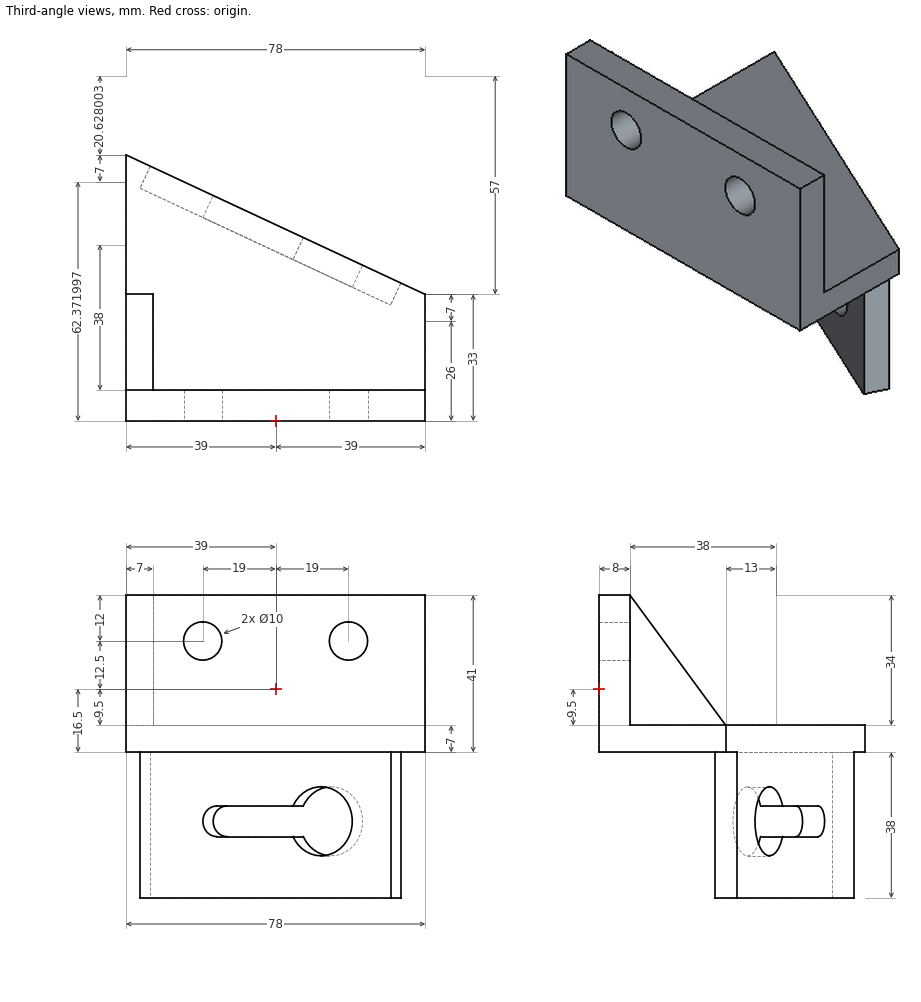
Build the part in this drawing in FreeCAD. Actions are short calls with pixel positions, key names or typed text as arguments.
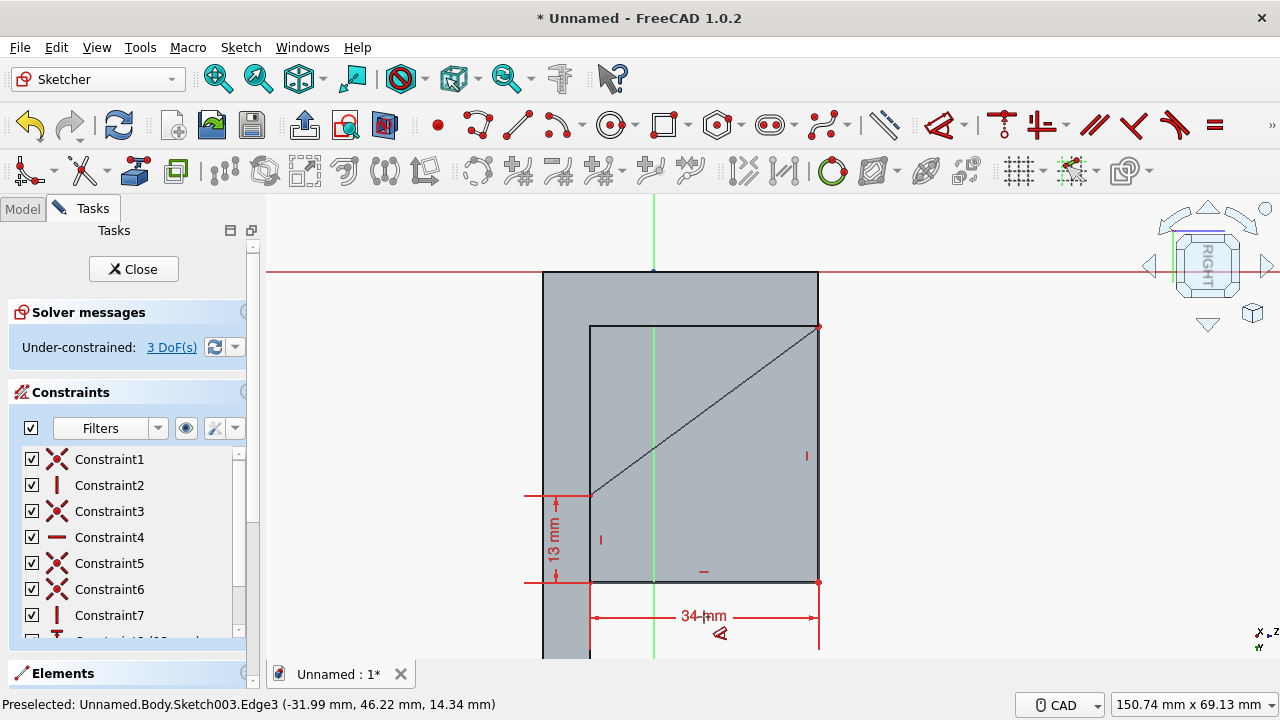
click(819, 506)
click(853, 455)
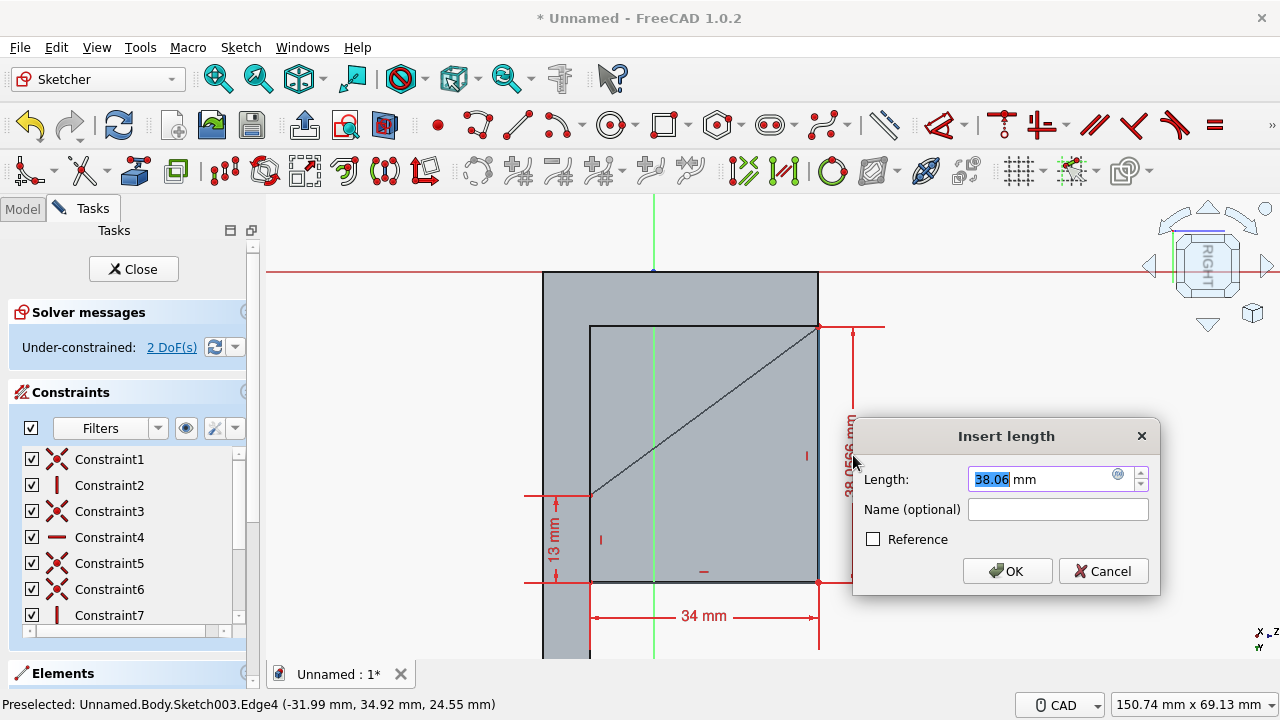
text(38)
key(Return)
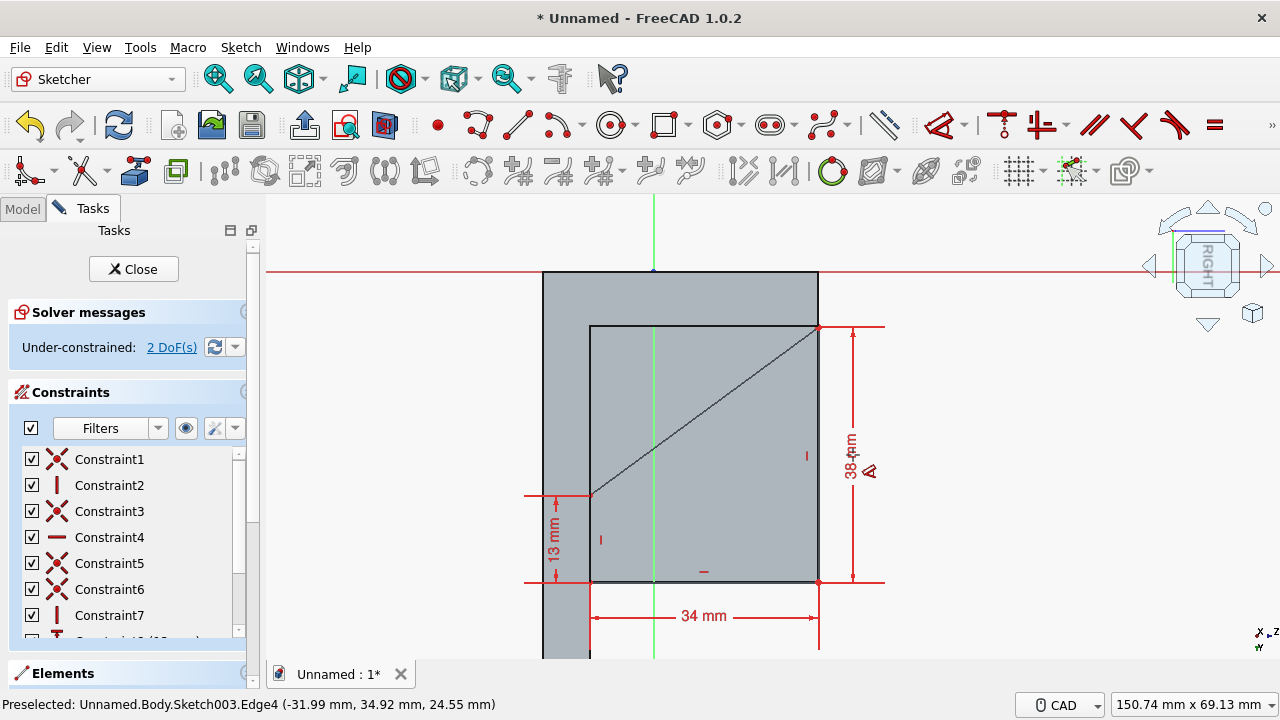
click(819, 327)
click(853, 300)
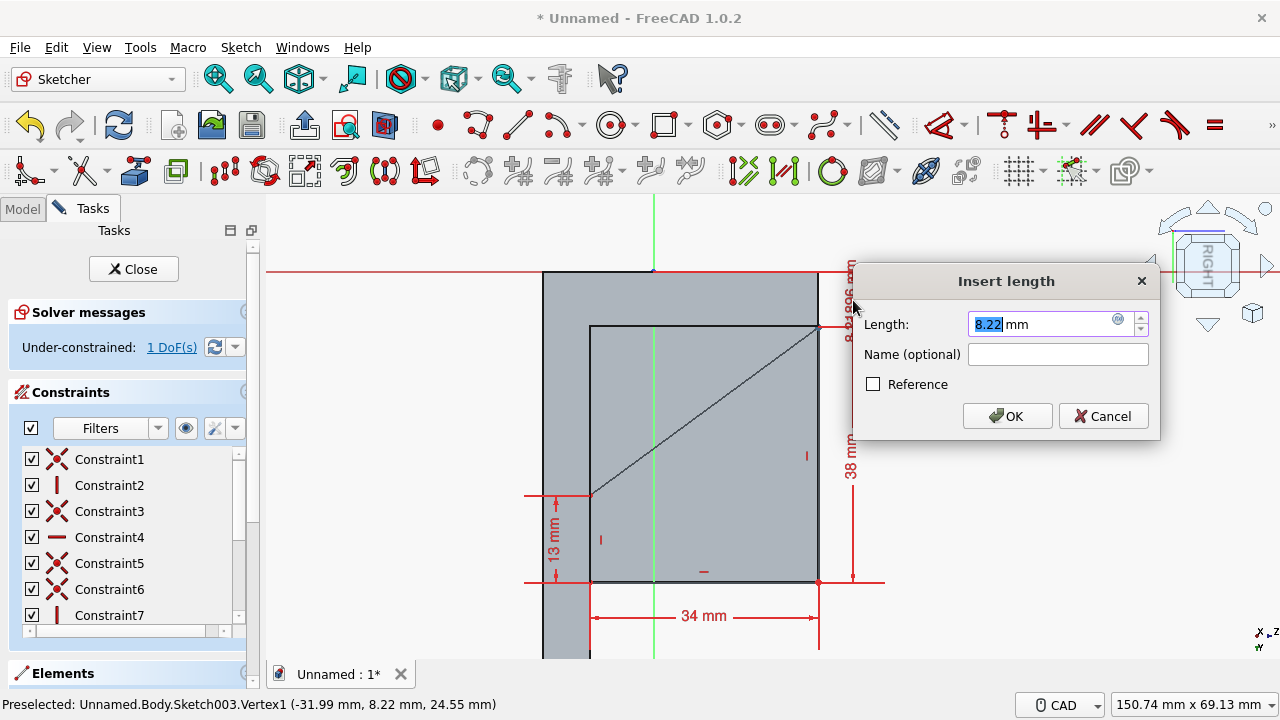
text(8)
key(Return)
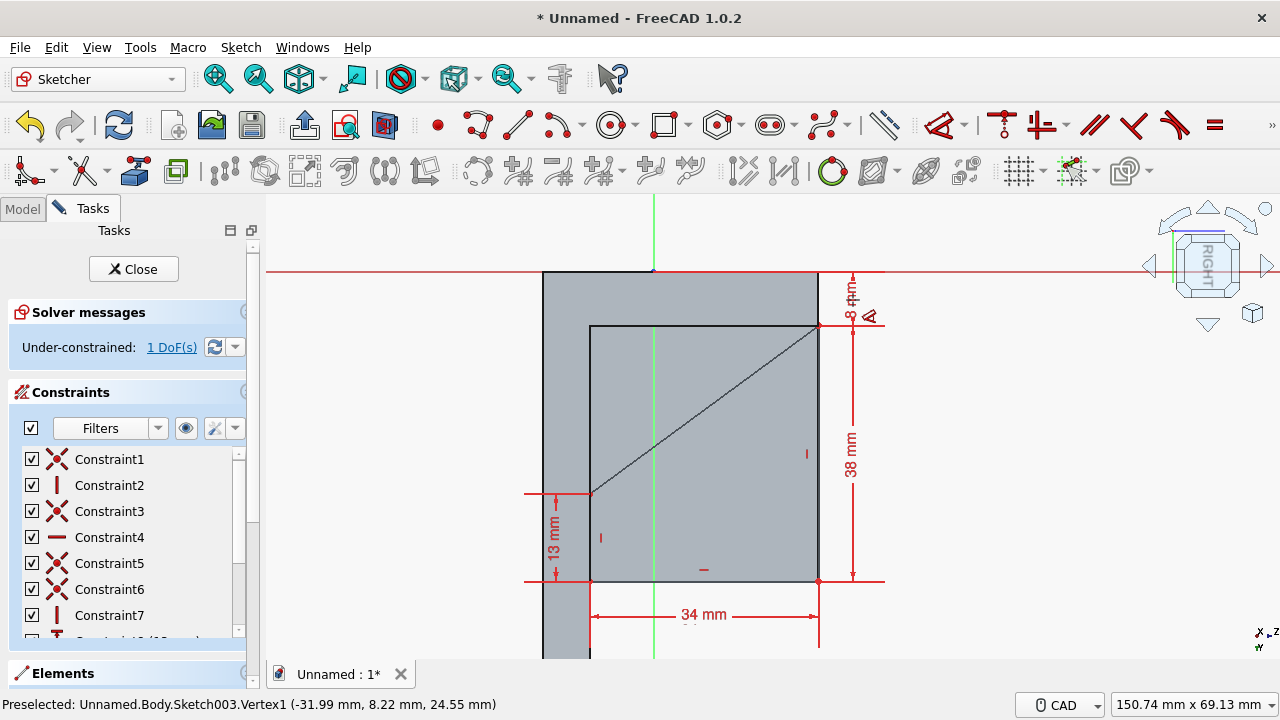
click(590, 494)
click(622, 238)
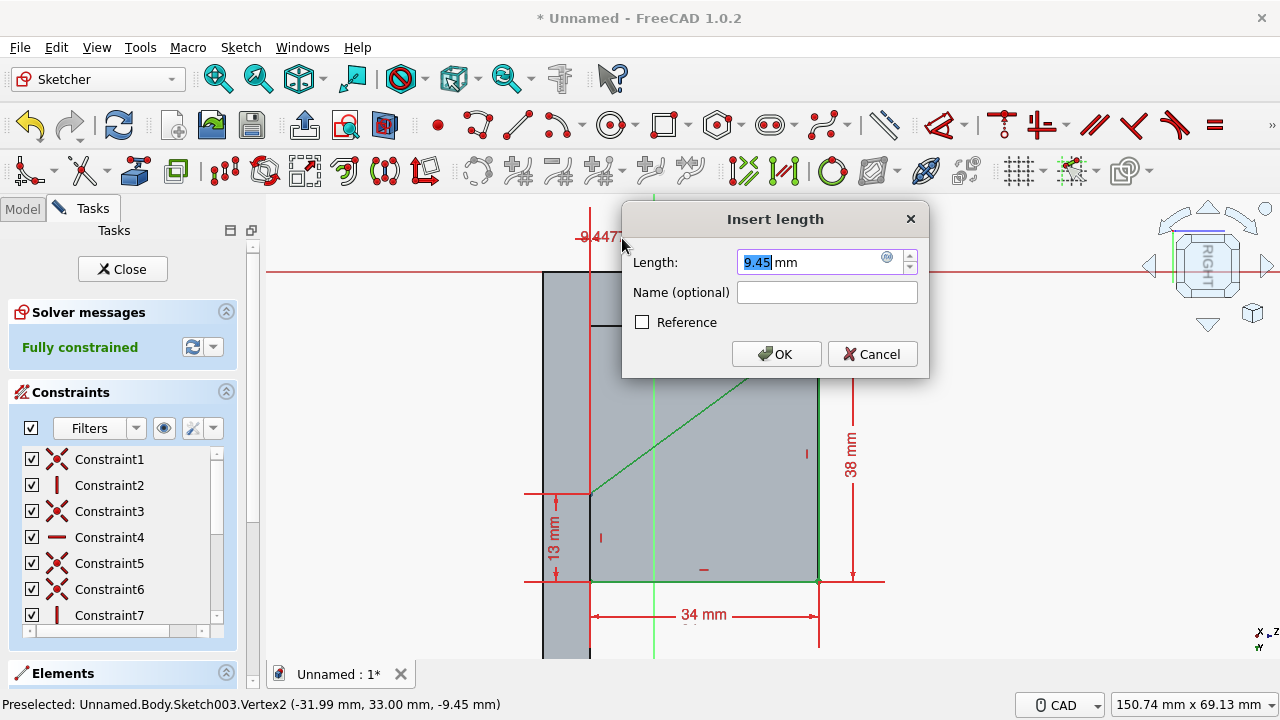
text(9.5)
key(Return)
key(Escape)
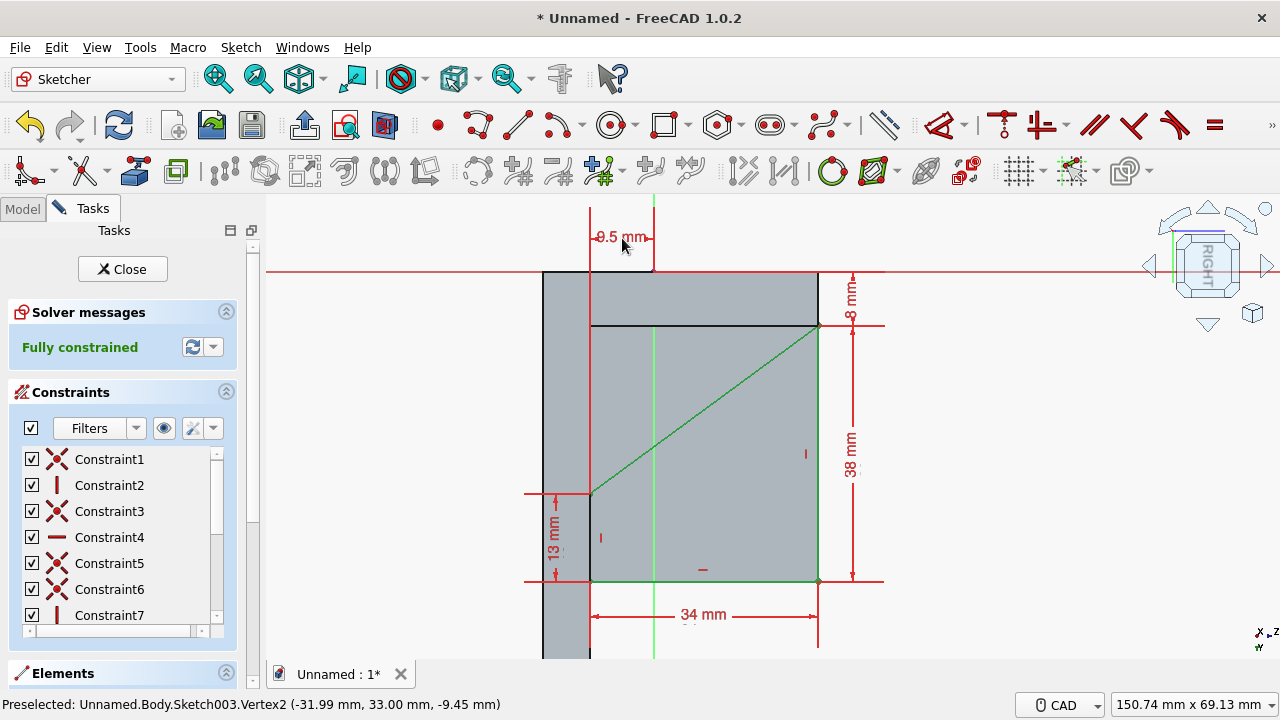
click(123, 269)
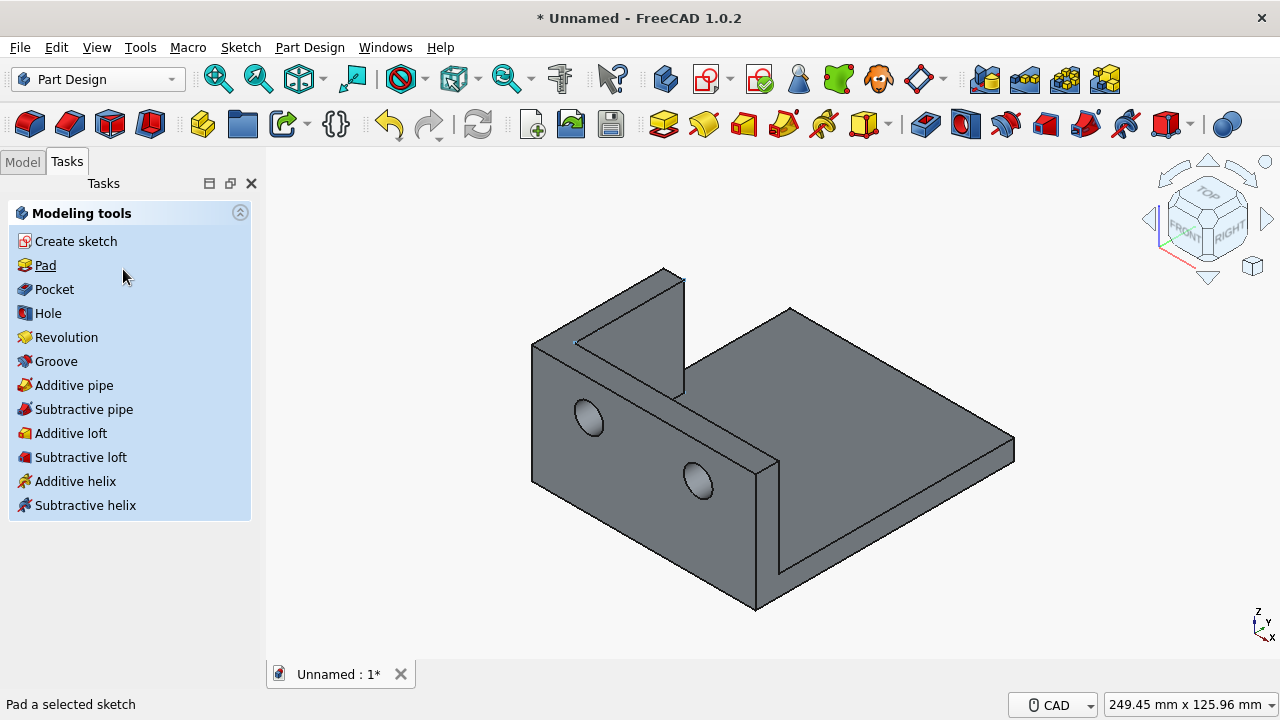
click(926, 124)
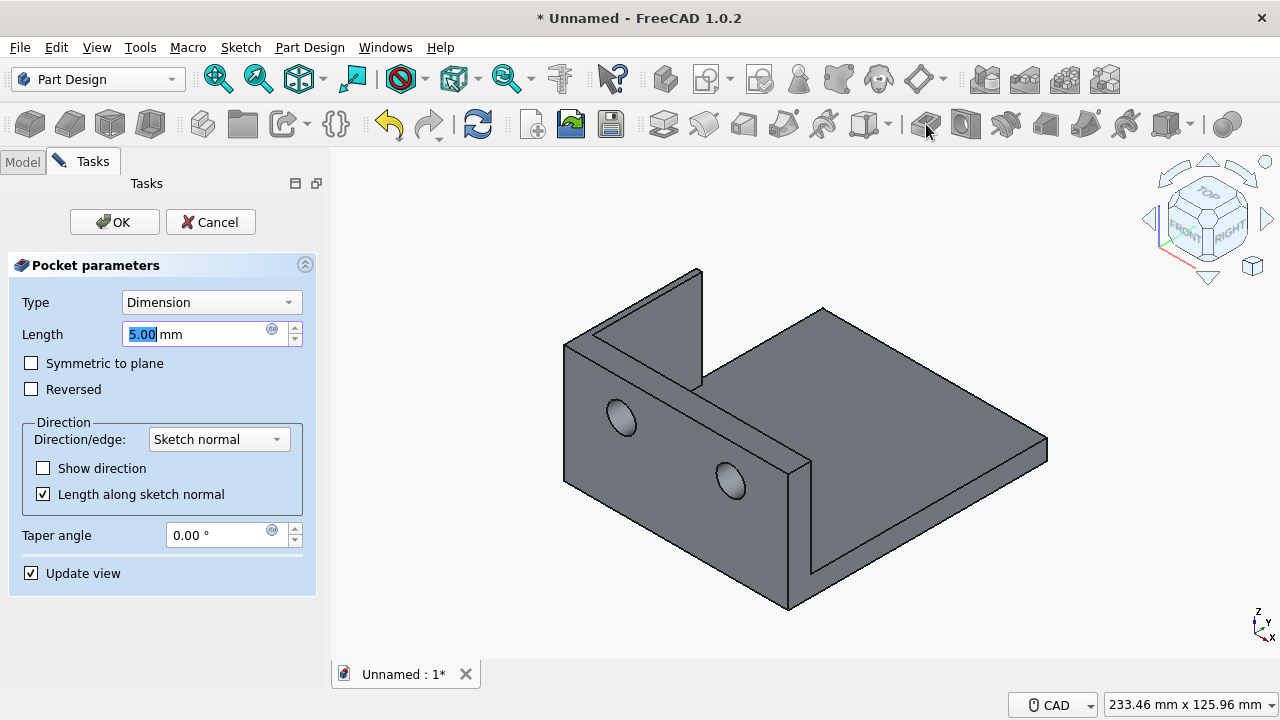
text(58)
key(Tab)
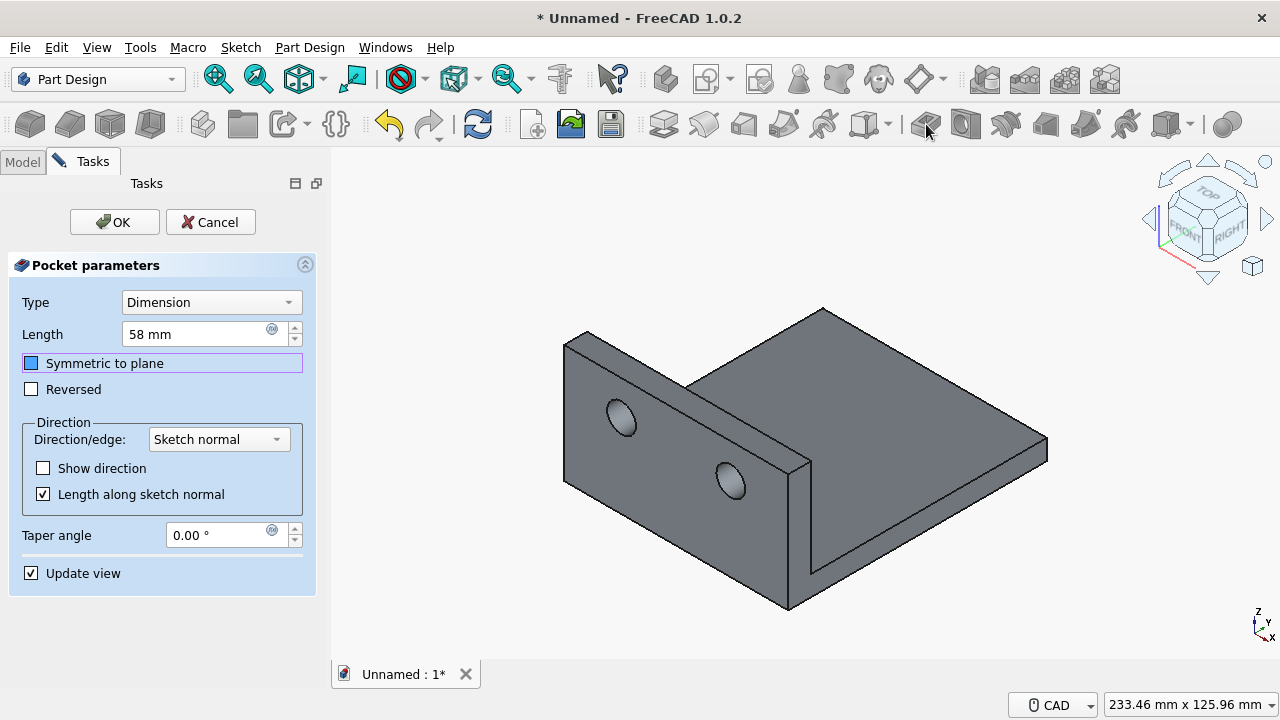
click(115, 222)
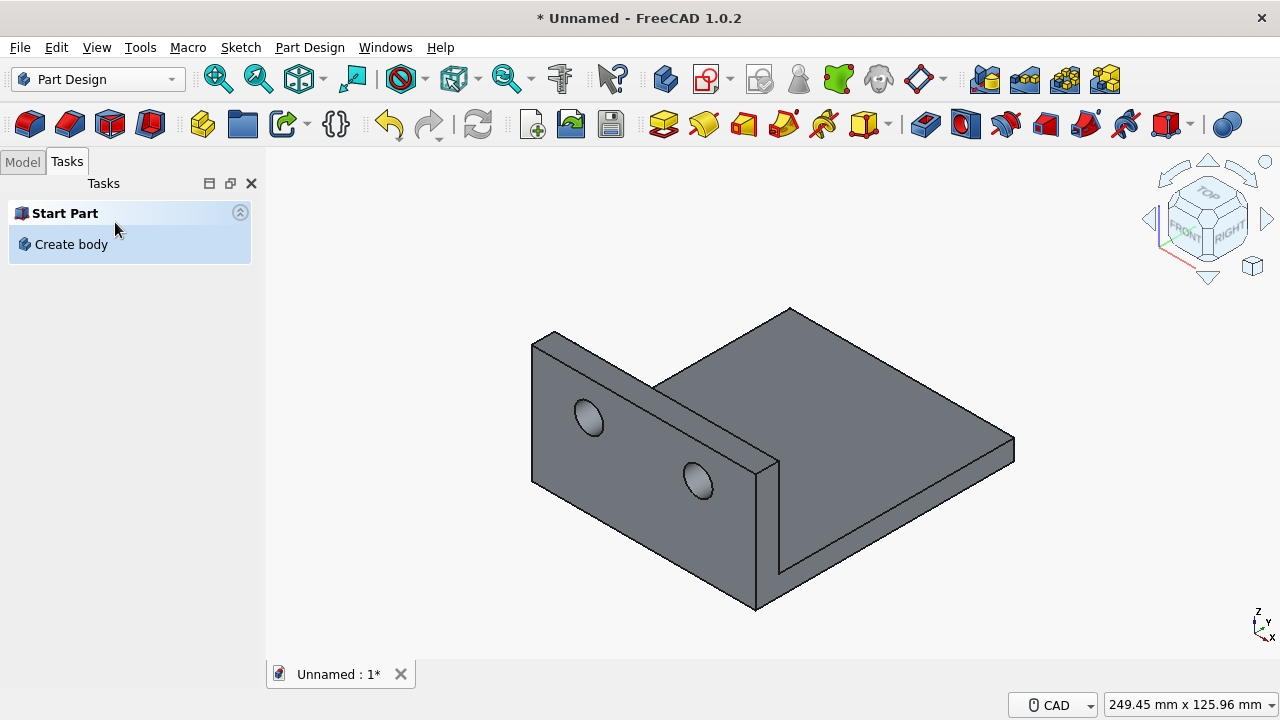
click(784, 440)